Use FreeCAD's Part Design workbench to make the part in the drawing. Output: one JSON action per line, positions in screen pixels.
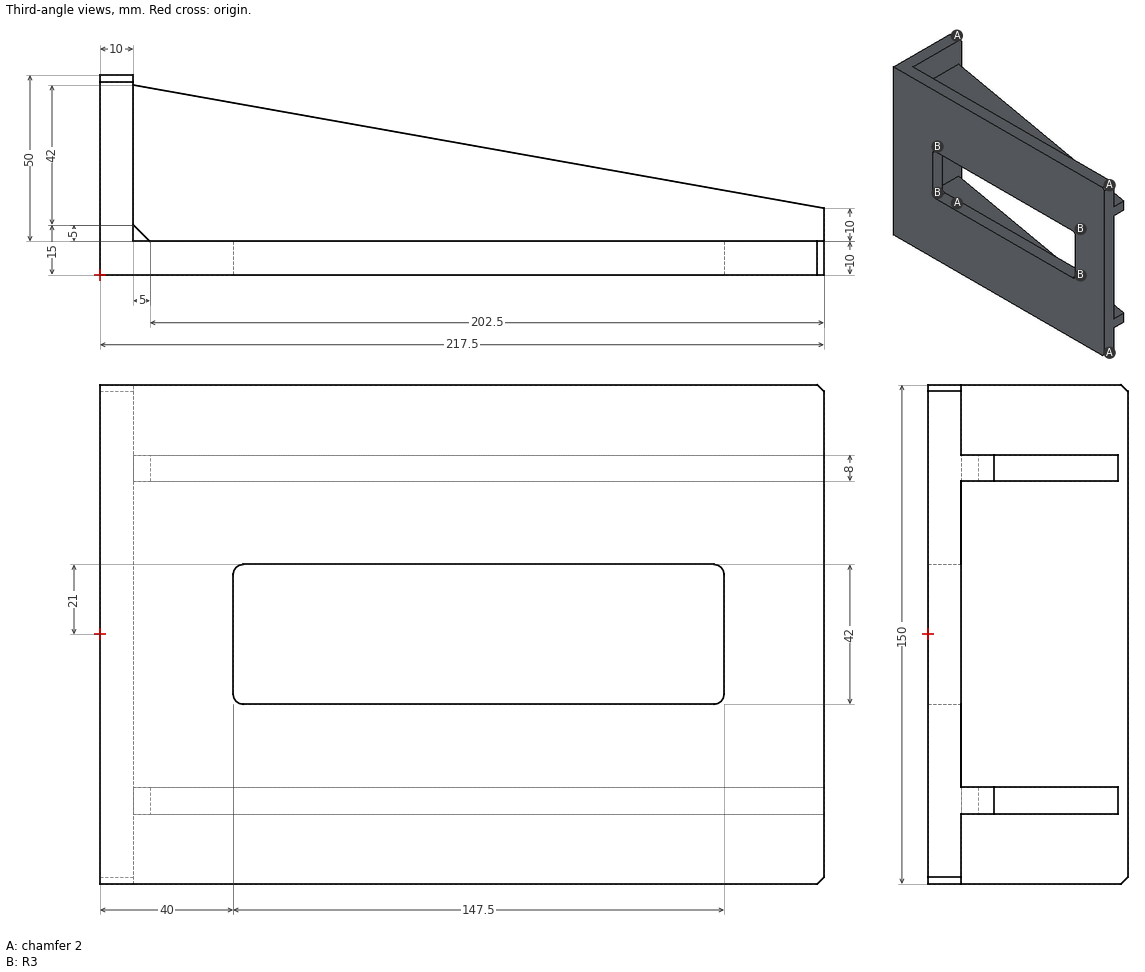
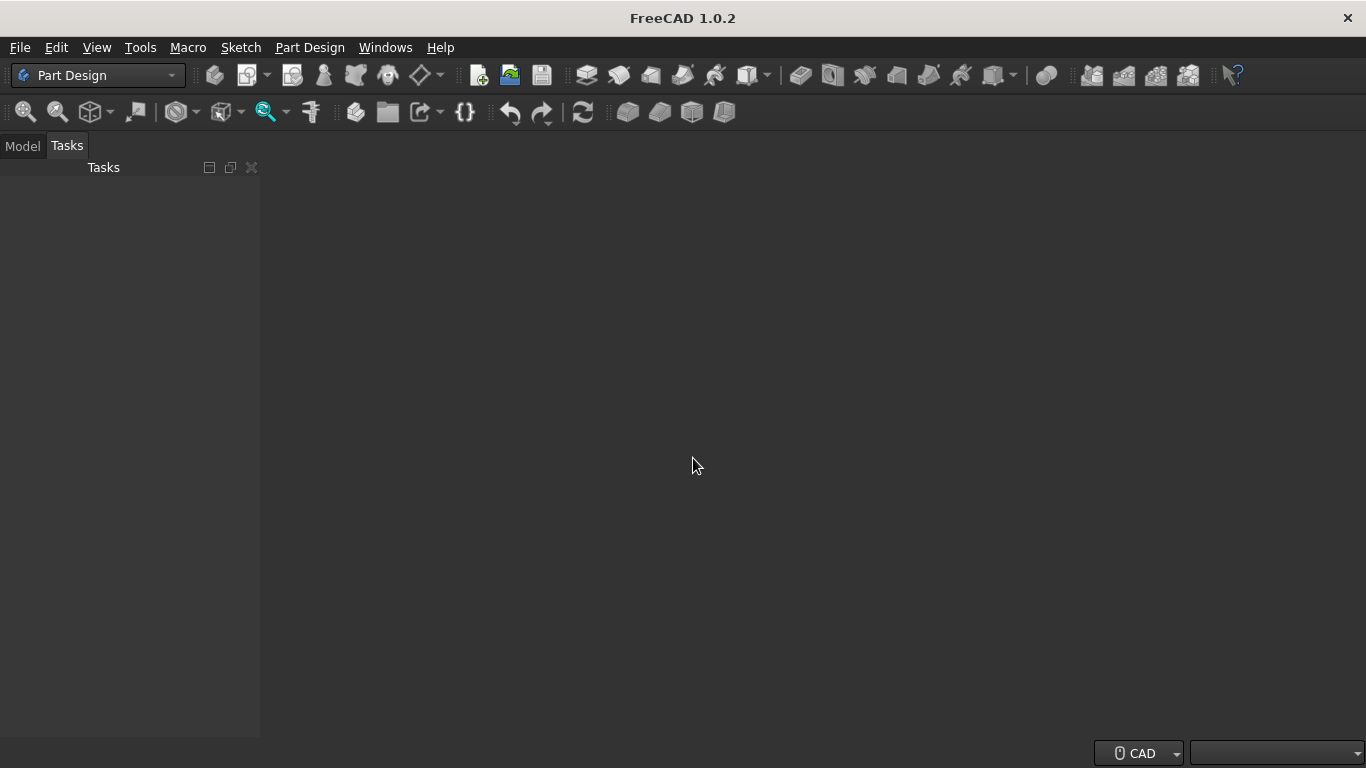
{"action": "left_click", "coordinate": [478, 76]}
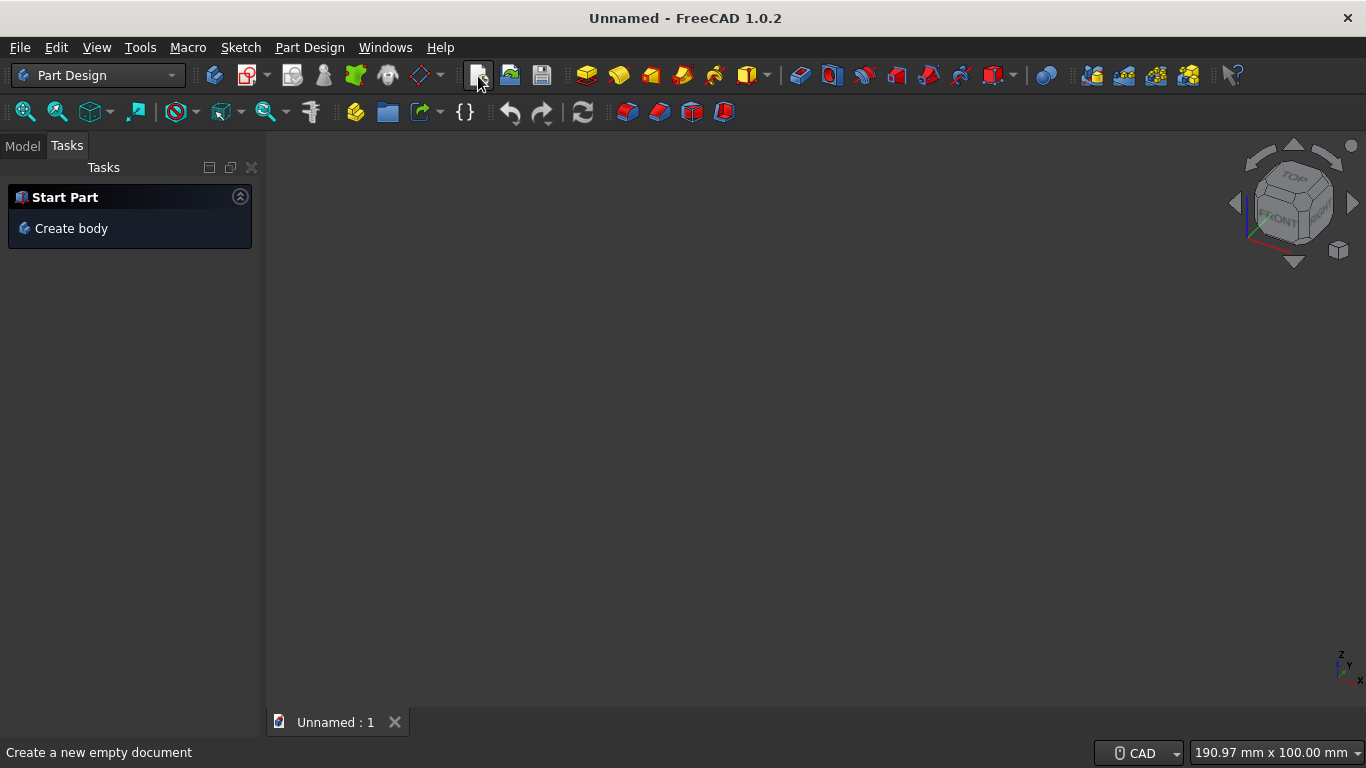
{"action": "left_click", "coordinate": [248, 76]}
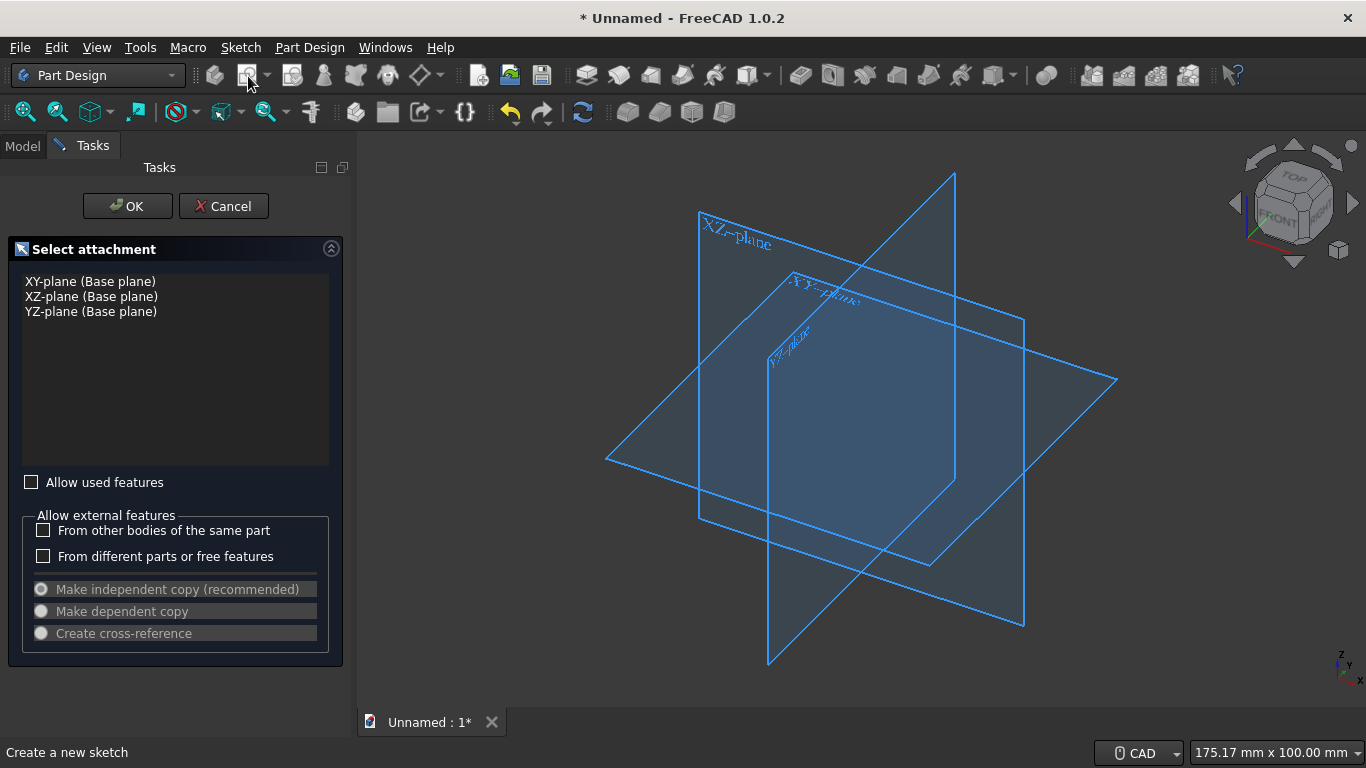
{"action": "left_click", "coordinate": [82, 282]}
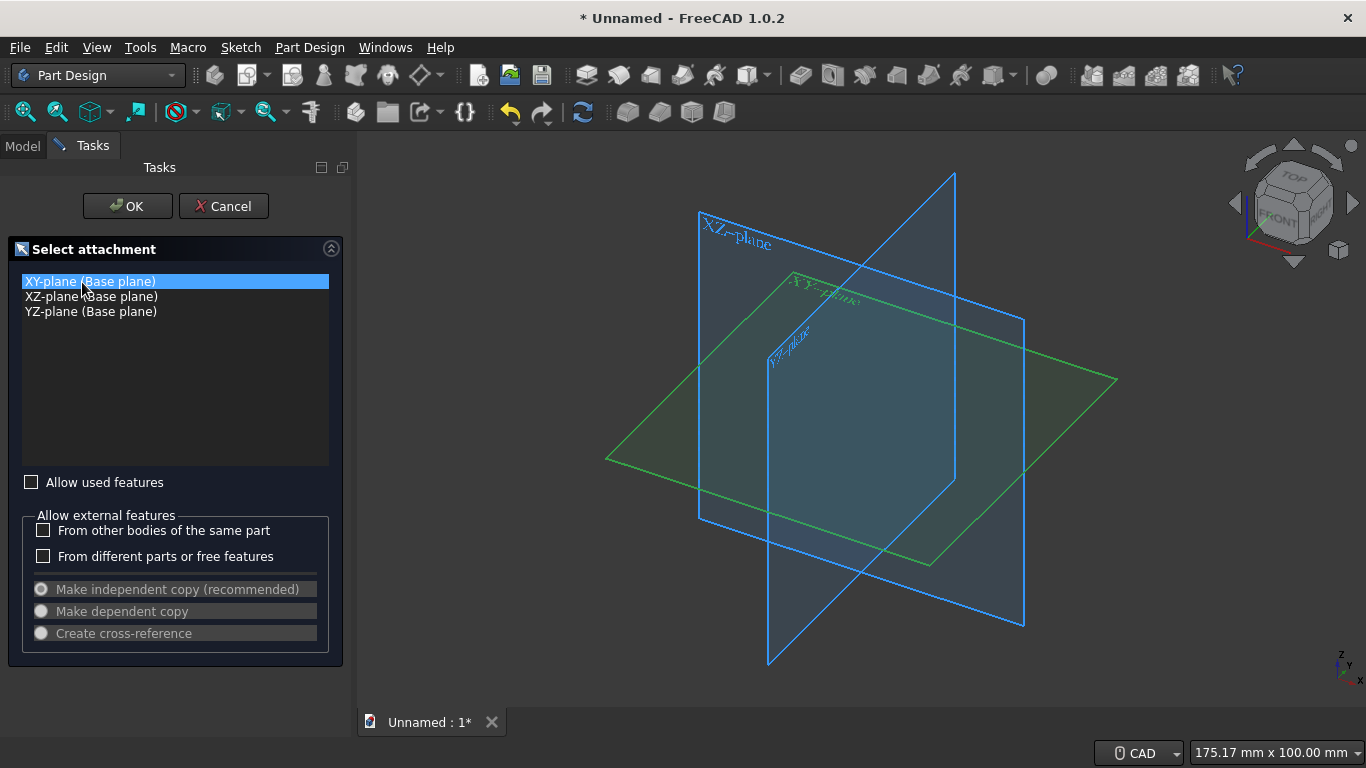
{"action": "left_click", "coordinate": [128, 206]}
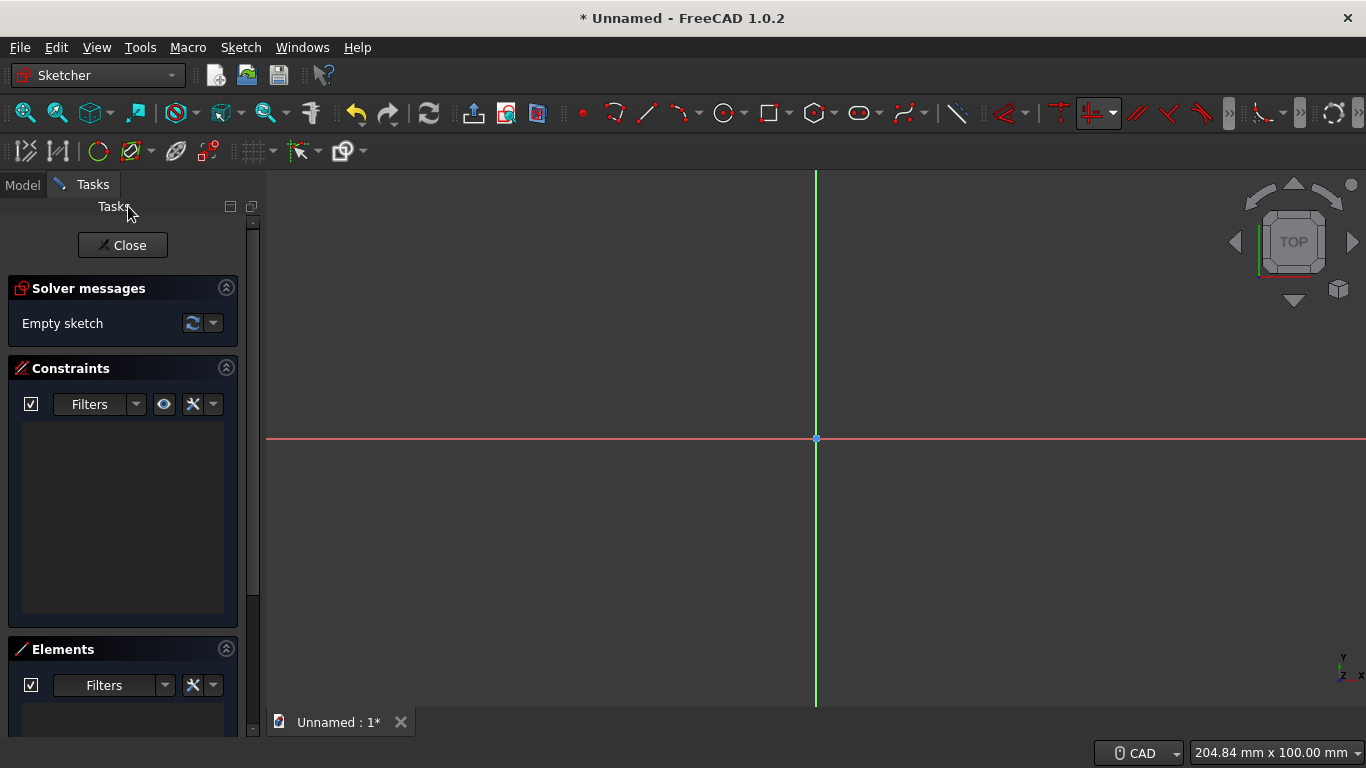
{"action": "scroll", "coordinate": [294, 570], "scroll_direction": "down", "scroll_amount": 4}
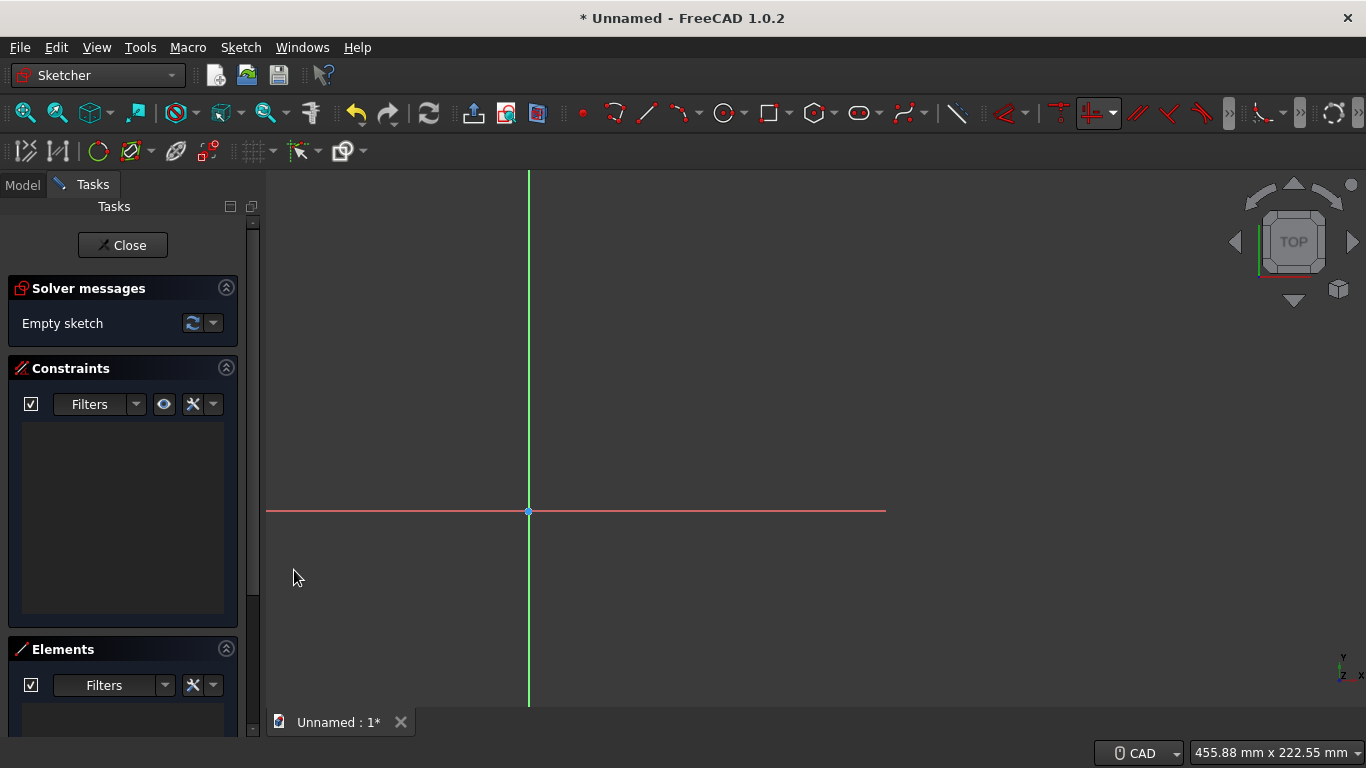
{"action": "left_click", "coordinate": [616, 114]}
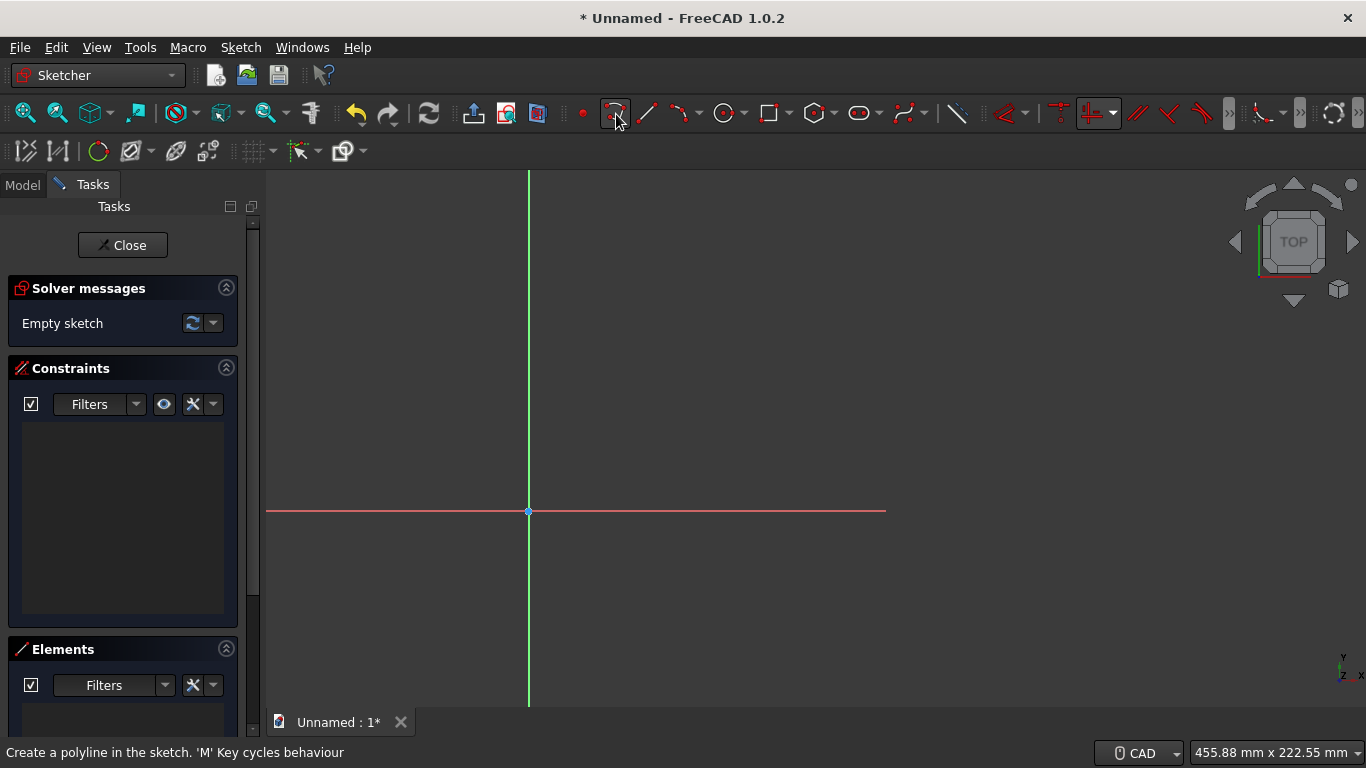
{"action": "left_click", "coordinate": [529, 511]}
{"action": "left_click", "coordinate": [1053, 502]}
{"action": "left_click", "coordinate": [1053, 487]}
{"action": "left_click", "coordinate": [553, 487]}
{"action": "left_click", "coordinate": [553, 367]}
{"action": "left_click", "coordinate": [538, 367]}
{"action": "left_click", "coordinate": [529, 511]}
{"action": "key", "text": "Escape"}
{"action": "key", "text": "Escape"}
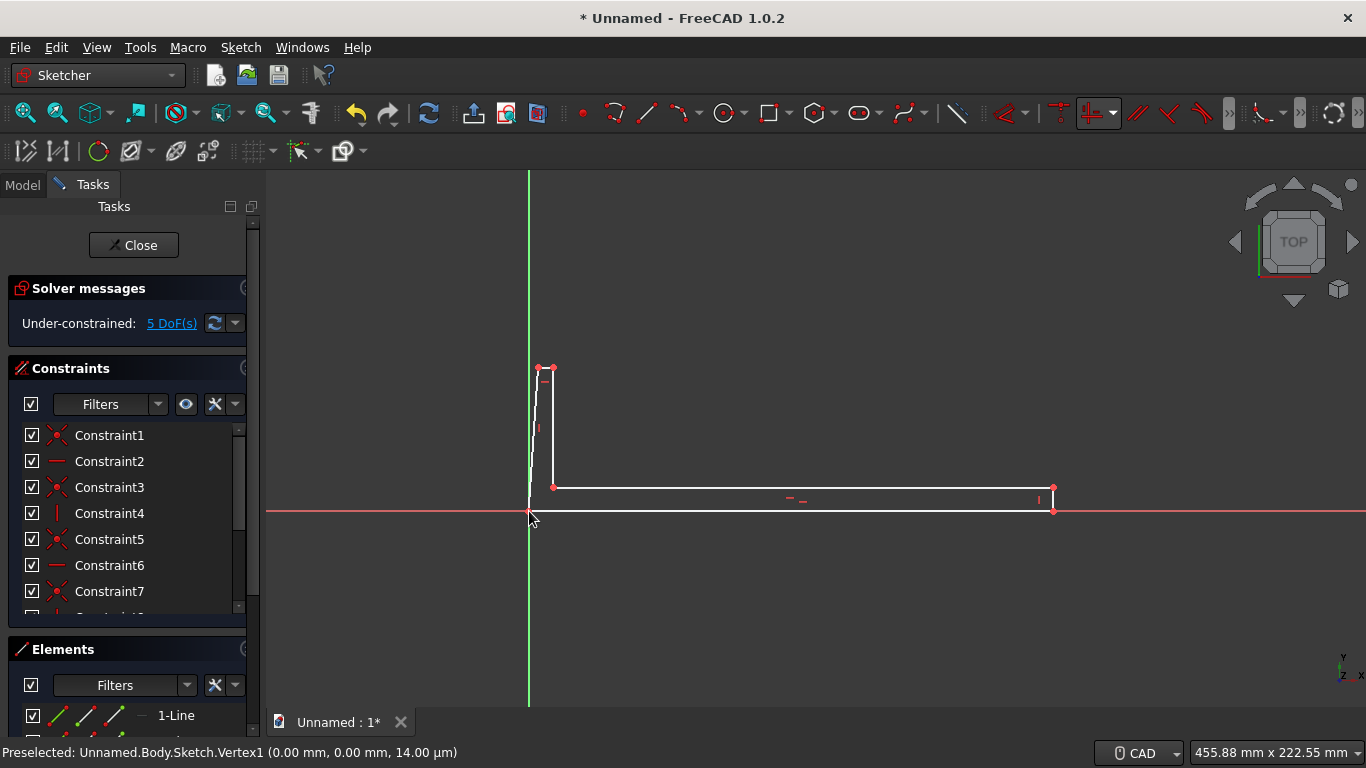
{"action": "left_click", "coordinate": [531, 468]}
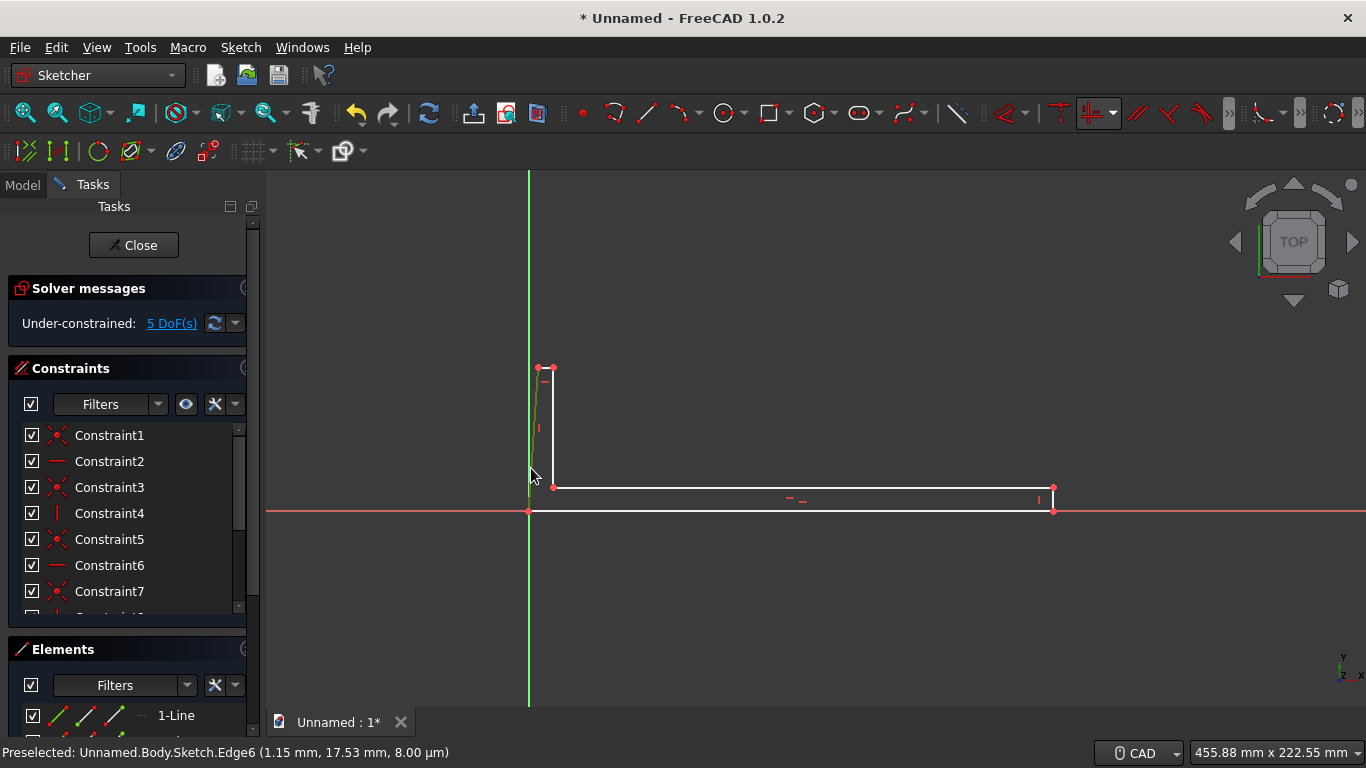
{"action": "key", "text": "v"}